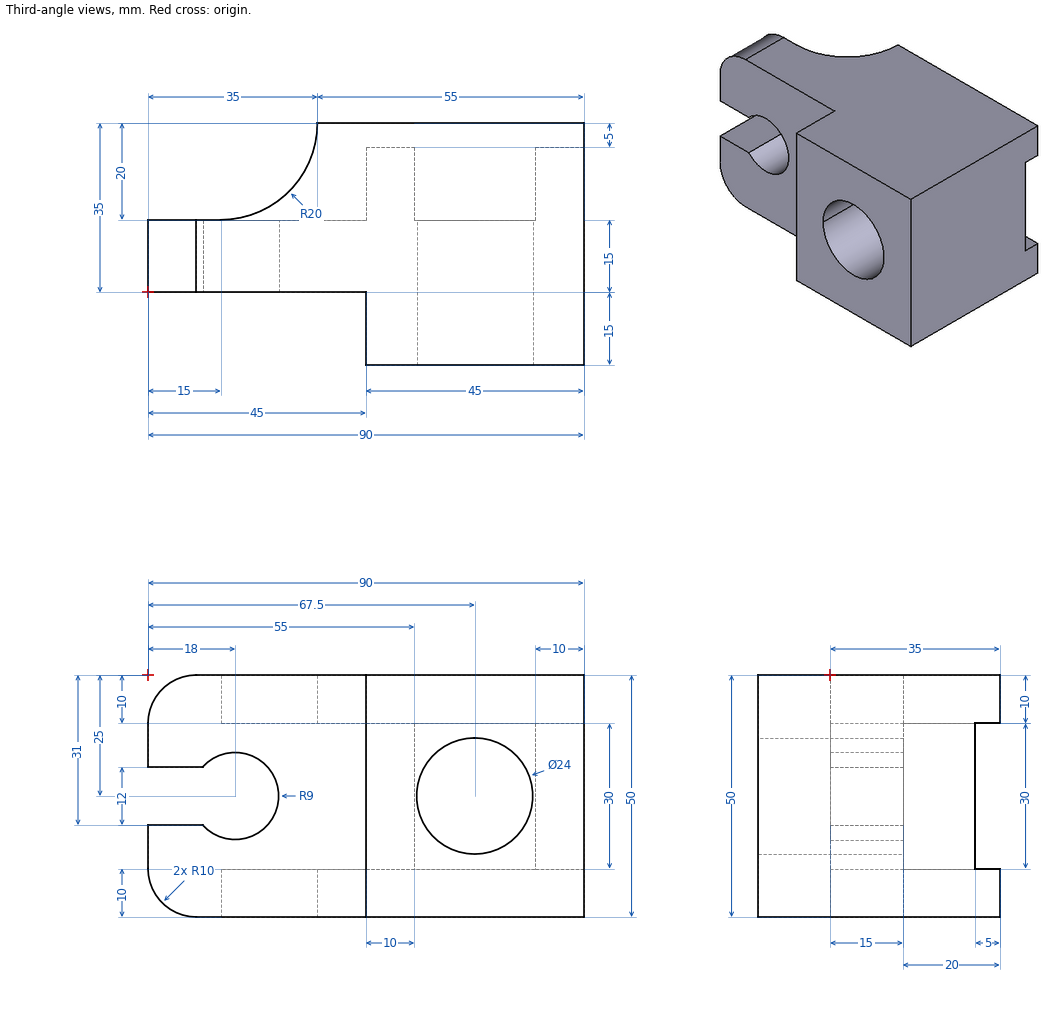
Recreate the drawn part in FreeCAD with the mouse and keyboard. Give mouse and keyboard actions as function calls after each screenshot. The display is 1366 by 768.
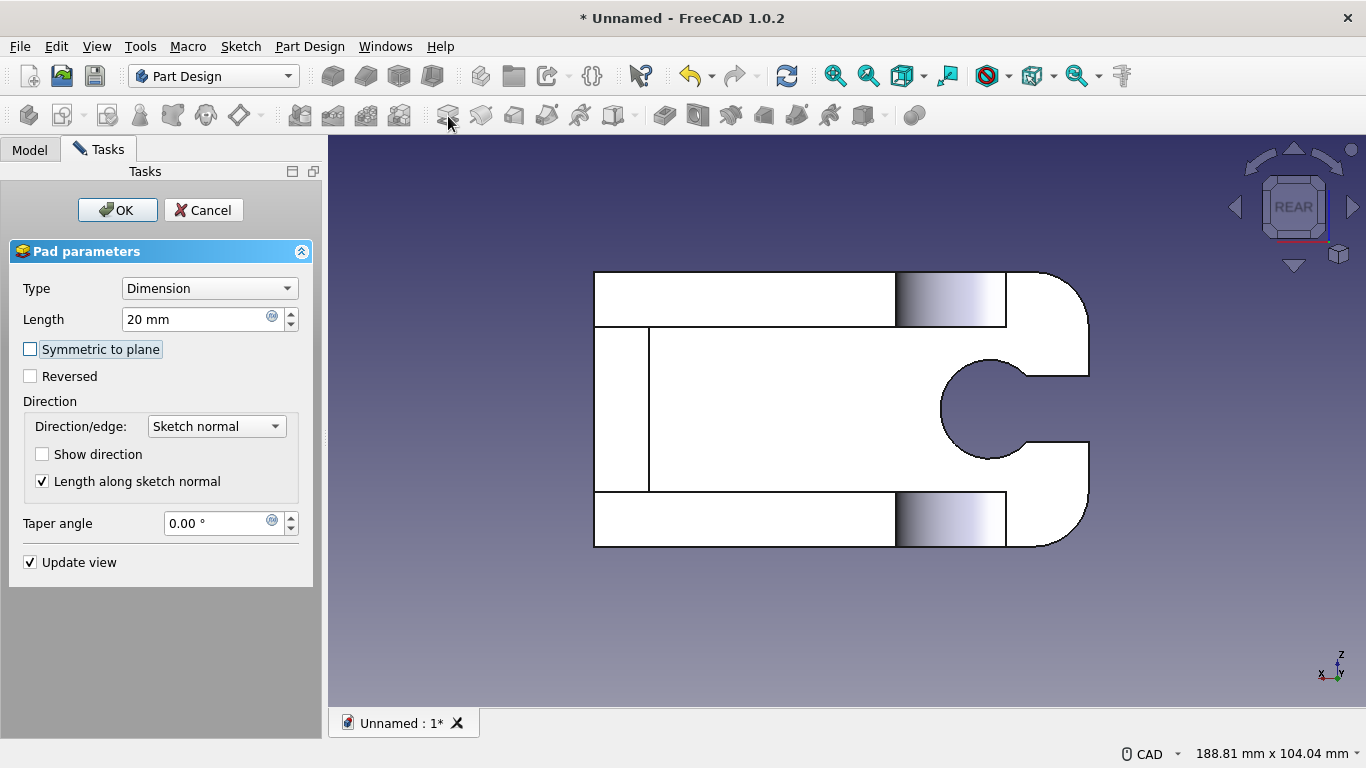
click(31, 376)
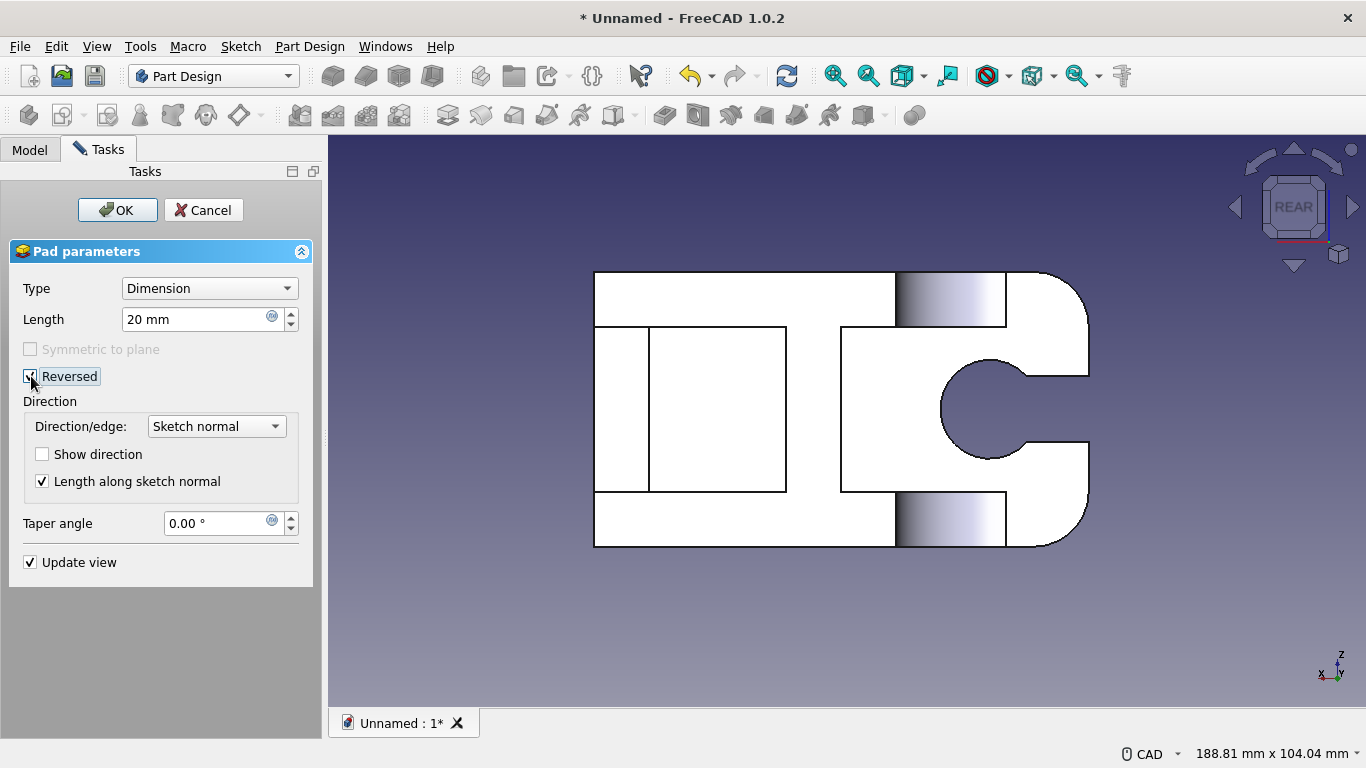
click(118, 210)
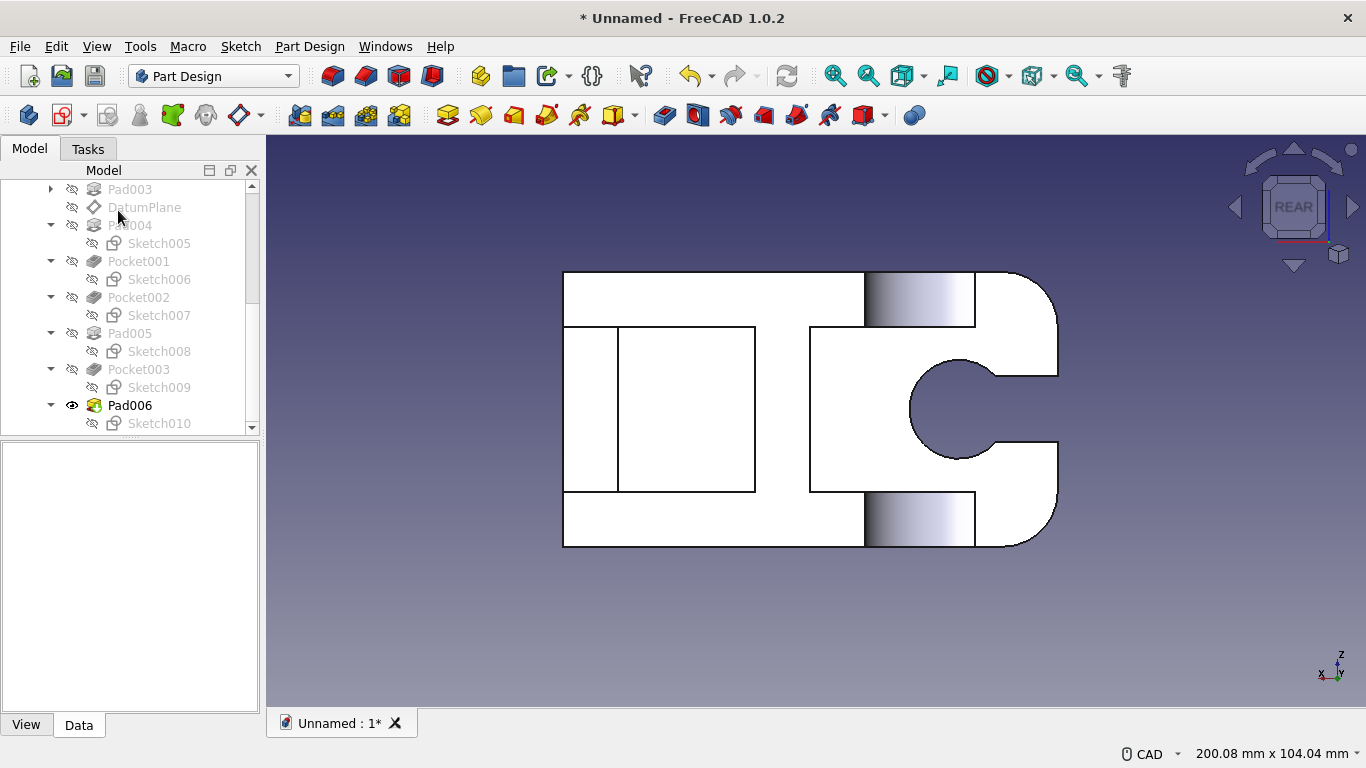
click(585, 290)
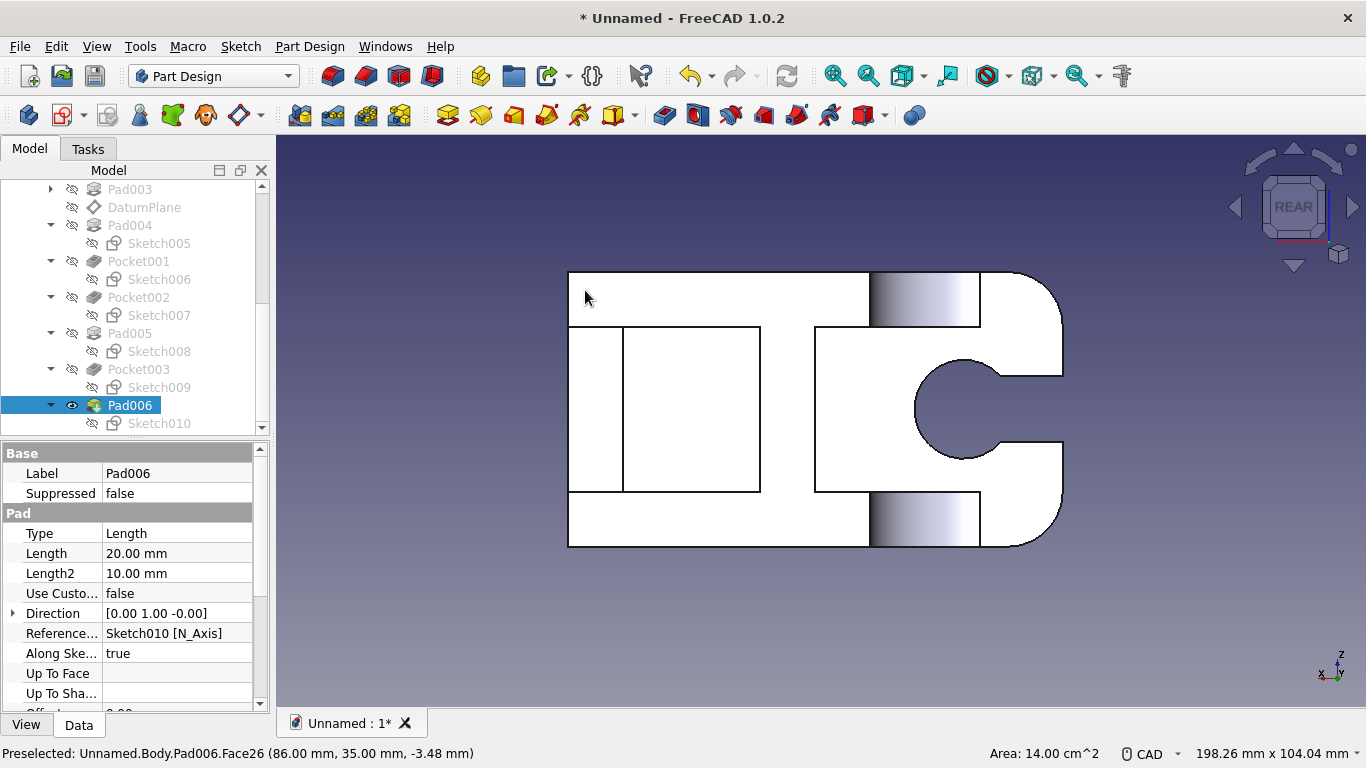
click(62, 116)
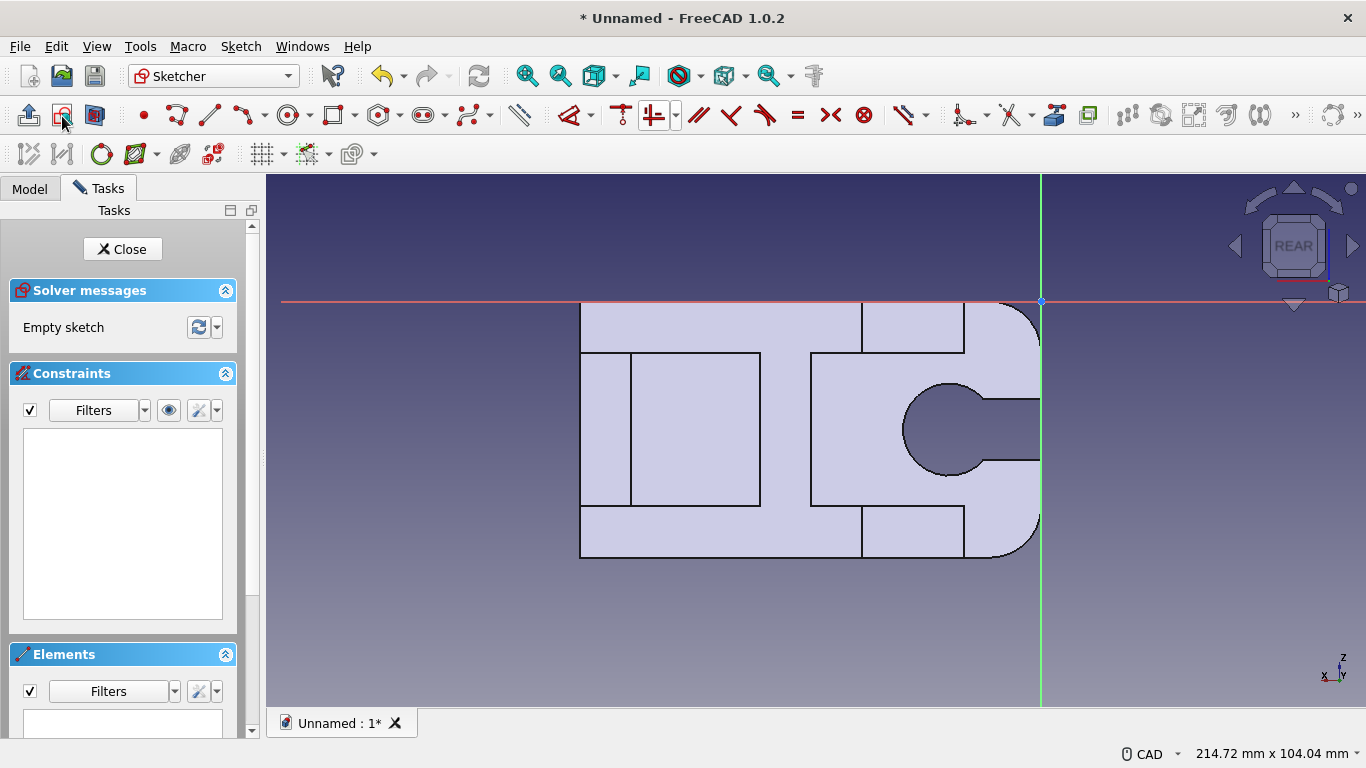
scroll(1201, 330, up, 2)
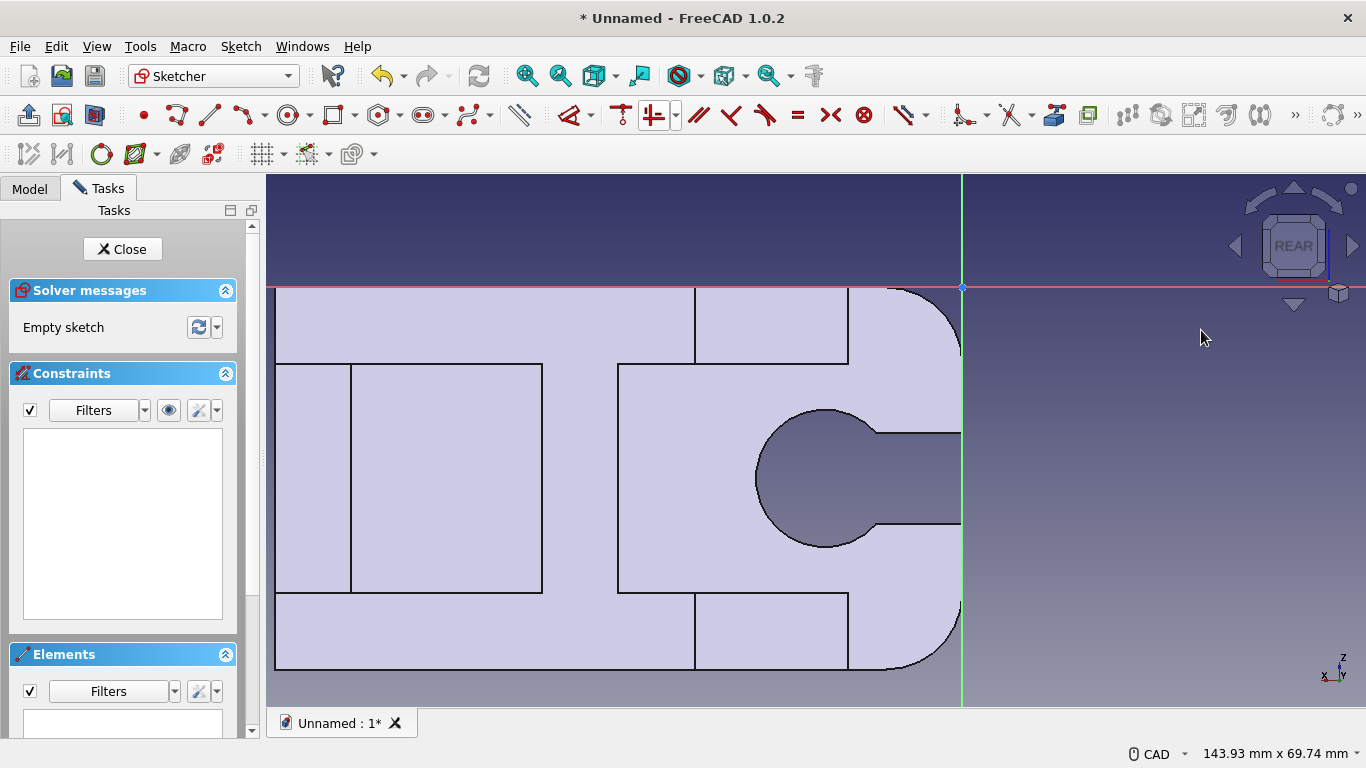
click(332, 116)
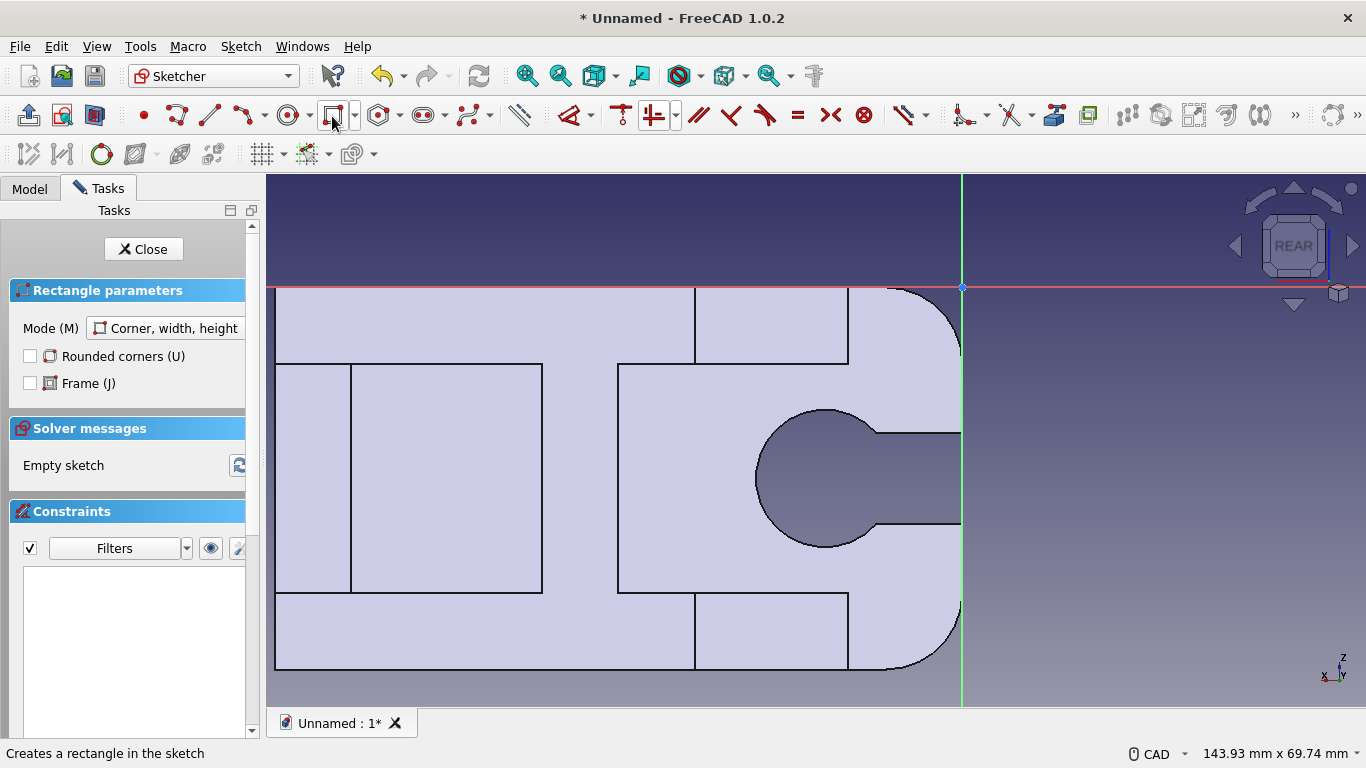
click(542, 364)
click(618, 593)
key(Escape)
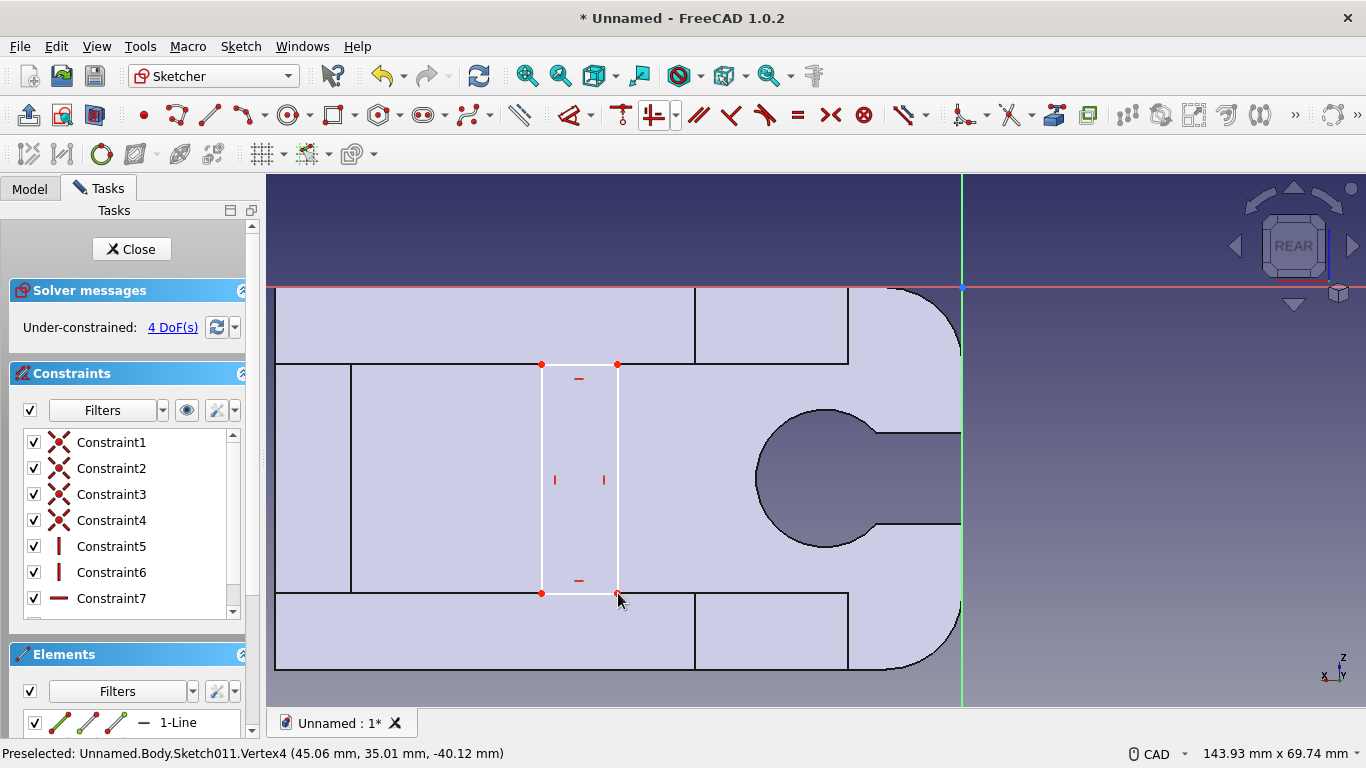
click(568, 116)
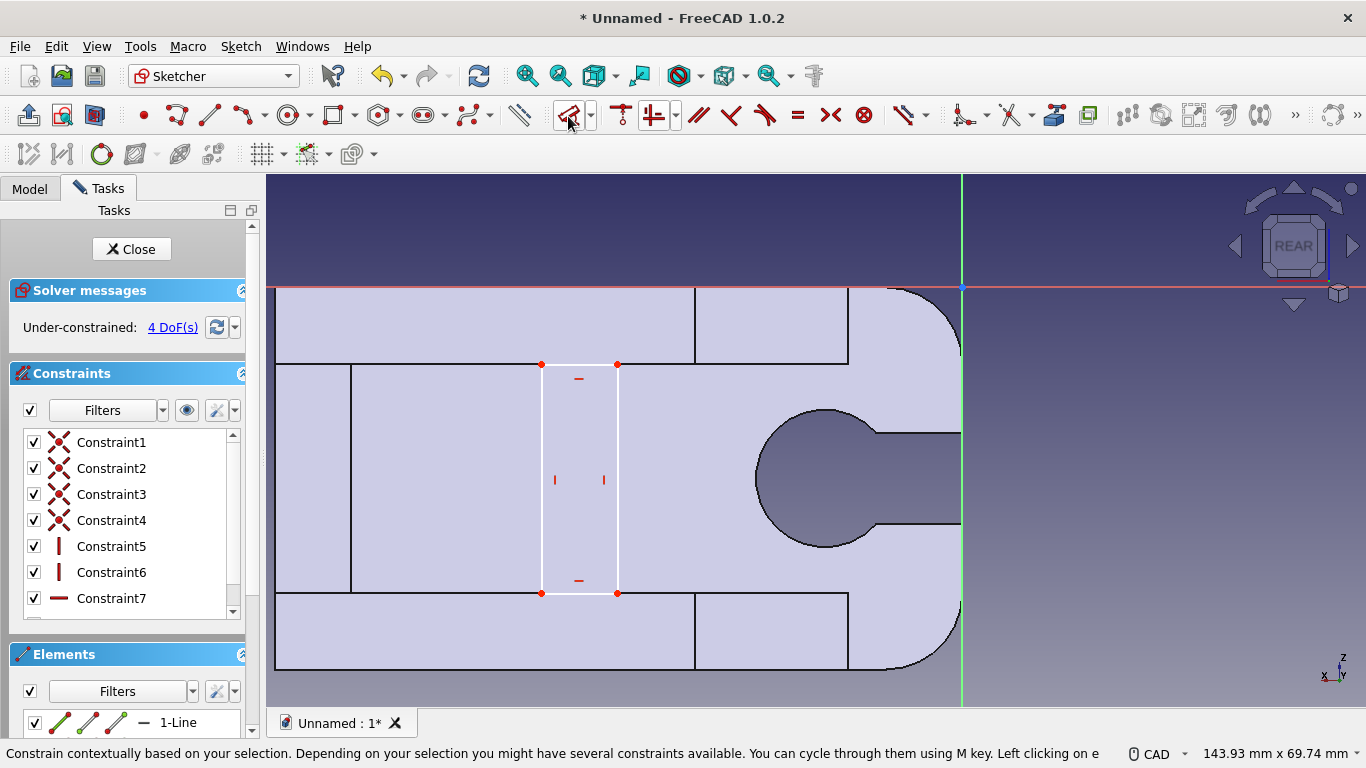
click(542, 434)
click(508, 480)